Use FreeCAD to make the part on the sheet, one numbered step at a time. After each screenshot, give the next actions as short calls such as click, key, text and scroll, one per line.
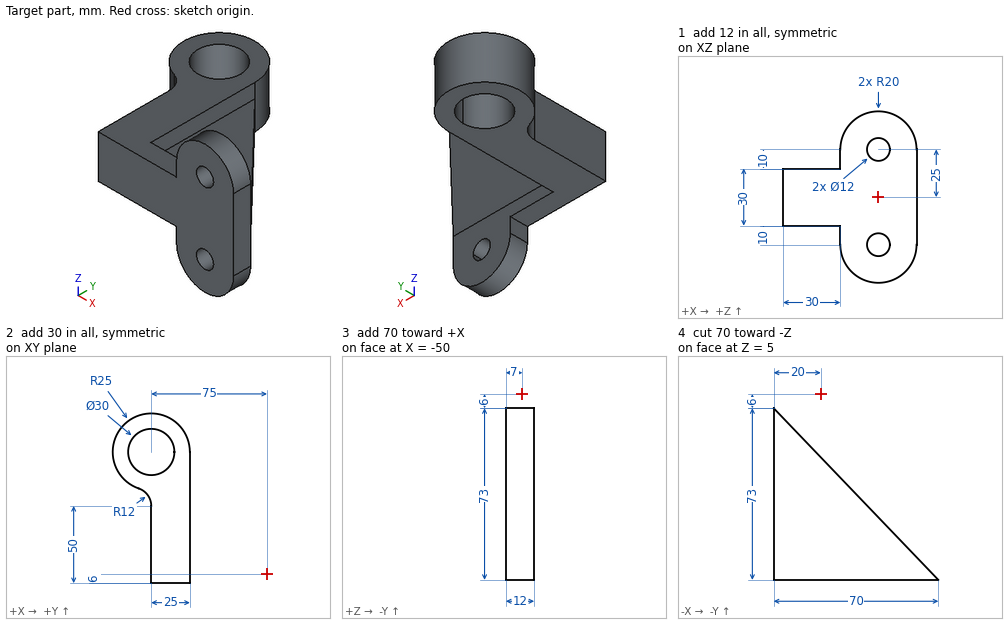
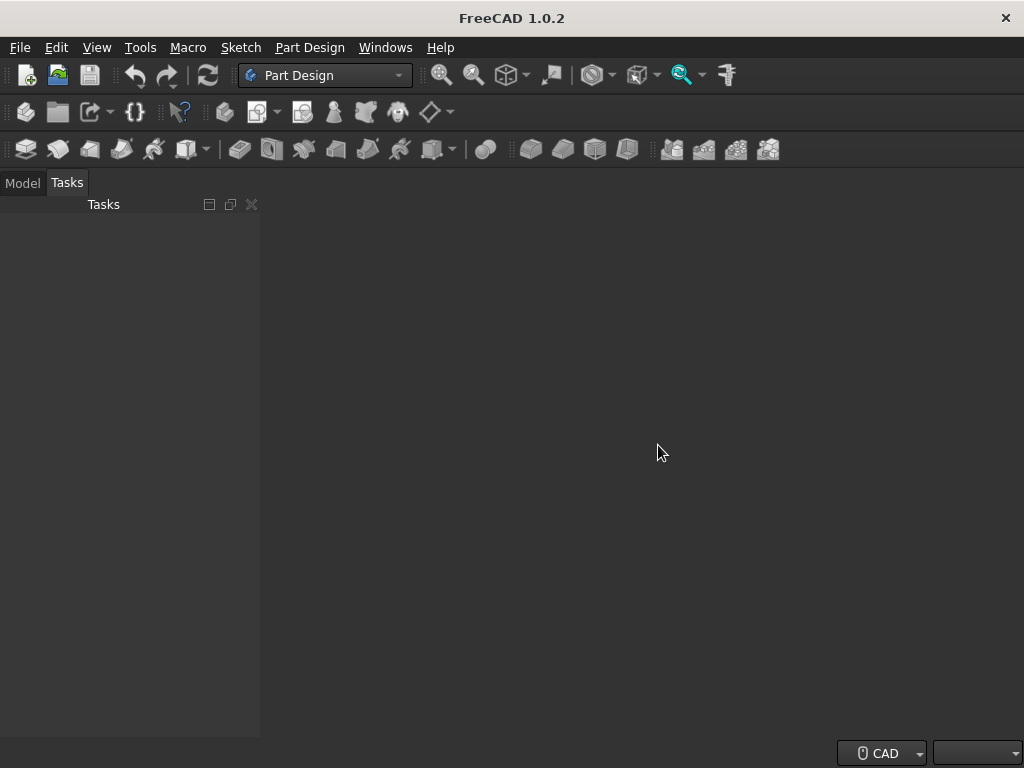
click(26, 76)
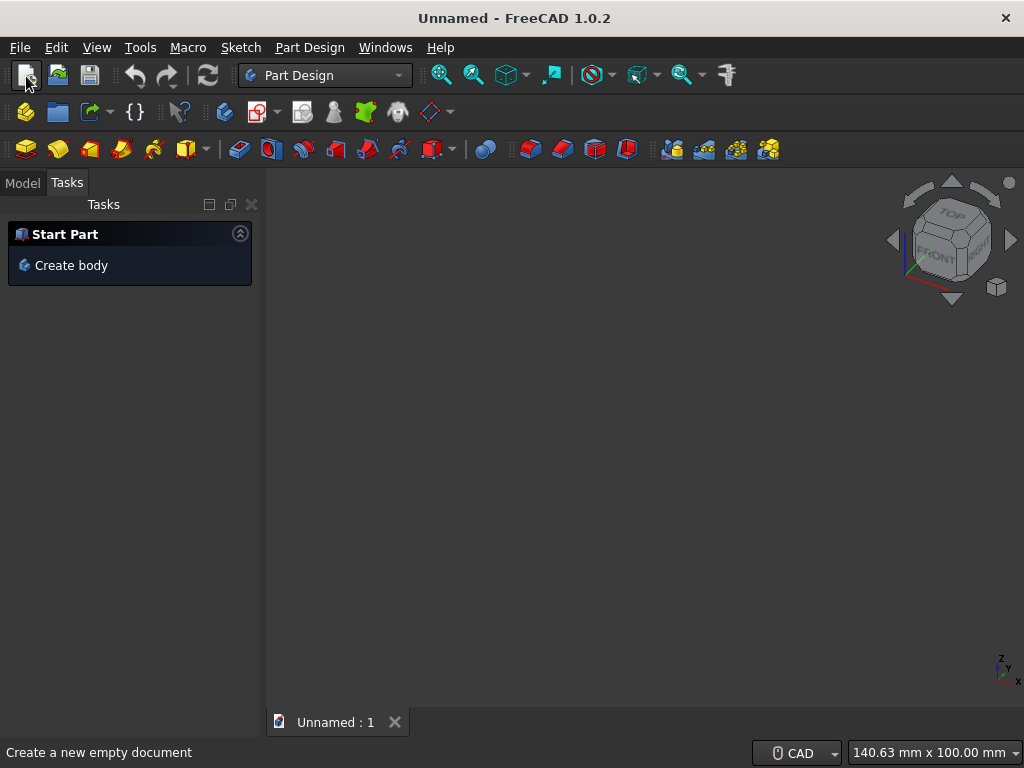
click(258, 112)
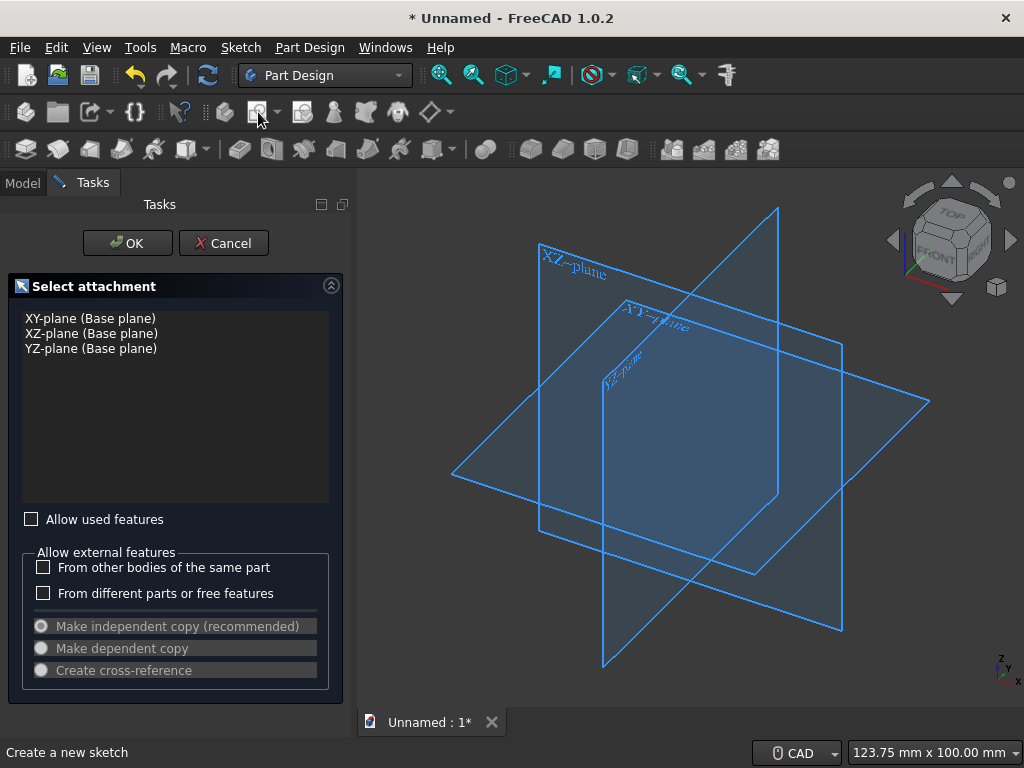
click(82, 334)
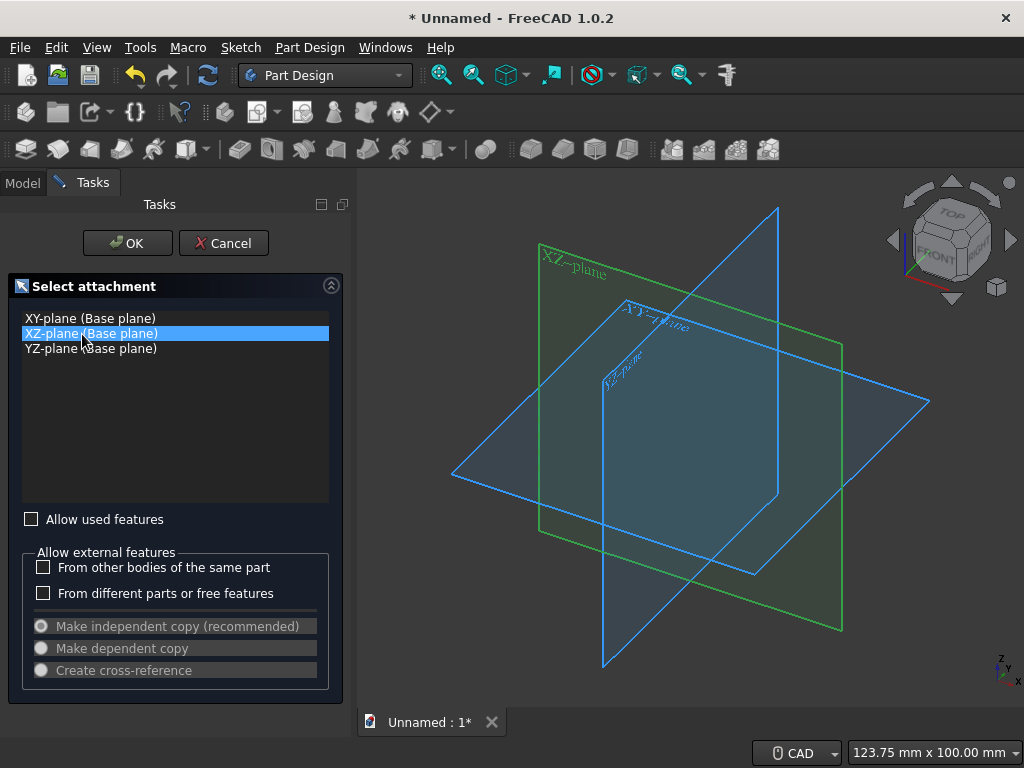
click(128, 243)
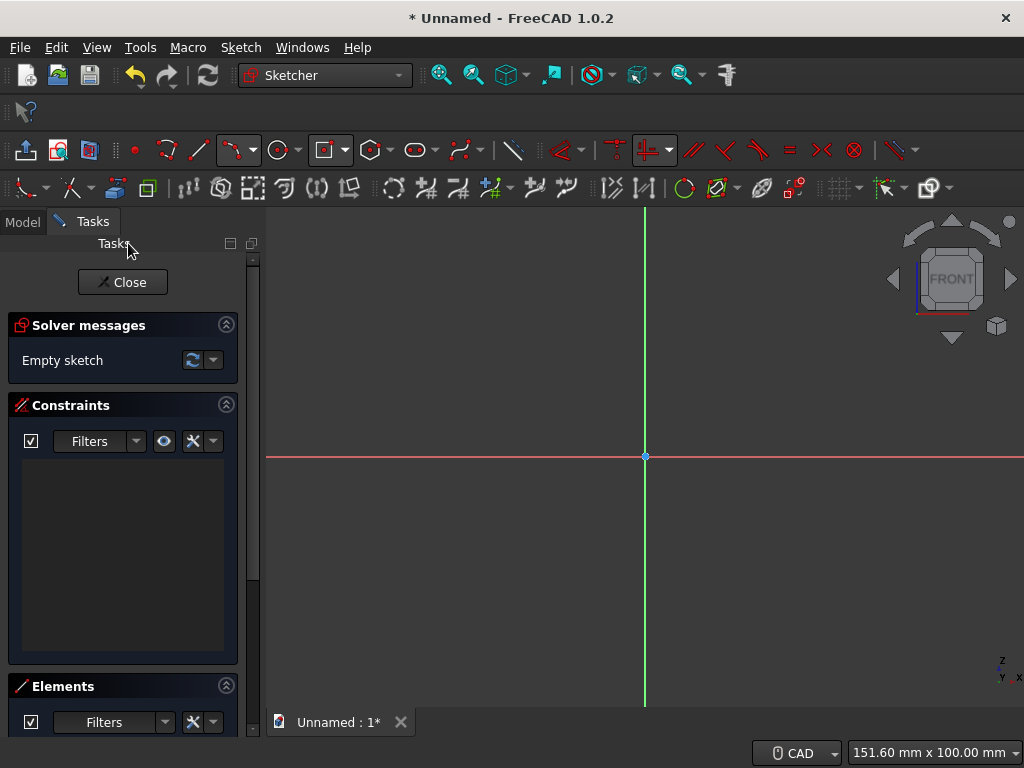
scroll(590, 457, down, 2)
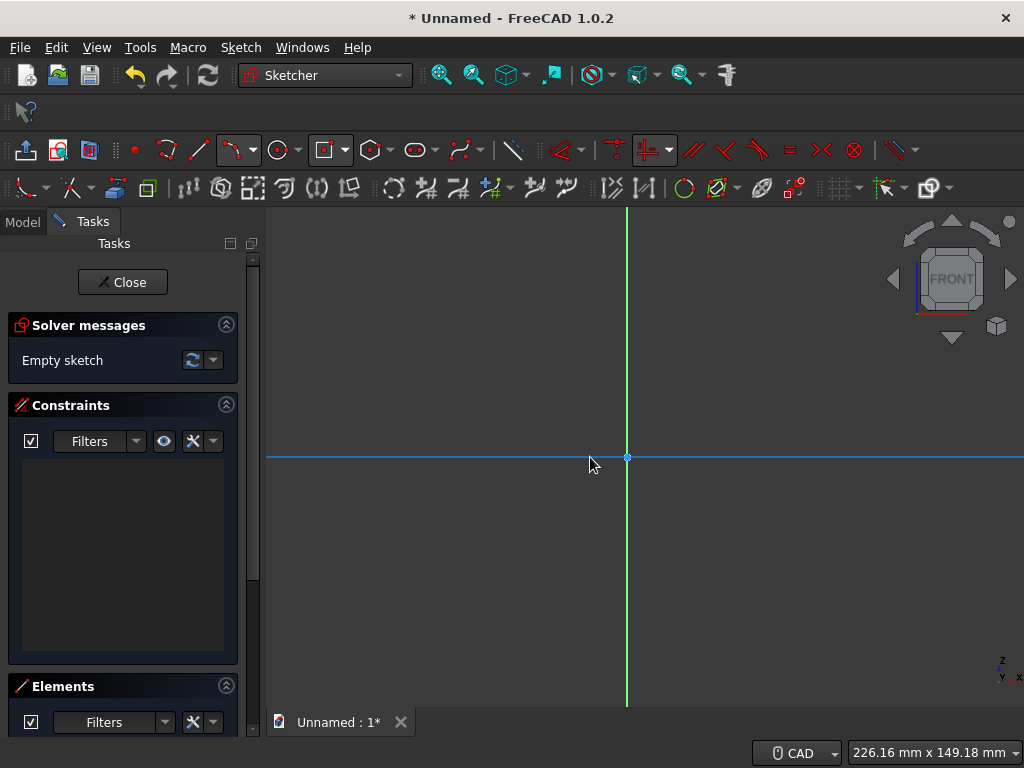
click(168, 150)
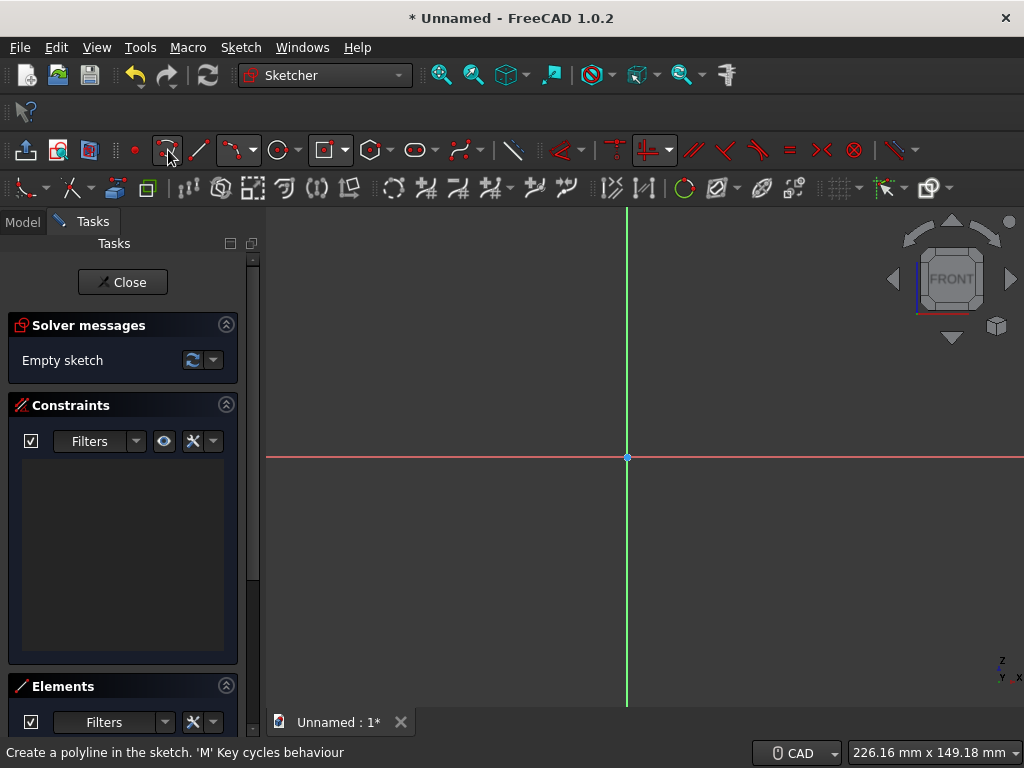
click(560, 541)
click(560, 507)
click(459, 507)
click(459, 407)
click(560, 407)
click(560, 373)
right_click(560, 373)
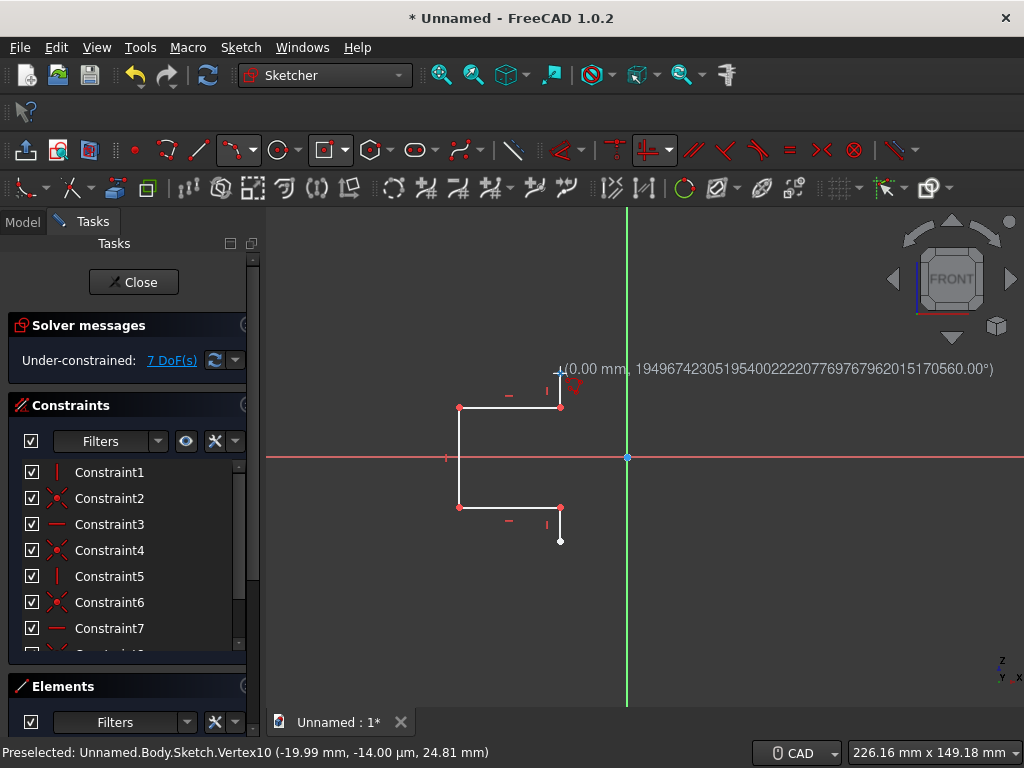
click(200, 150)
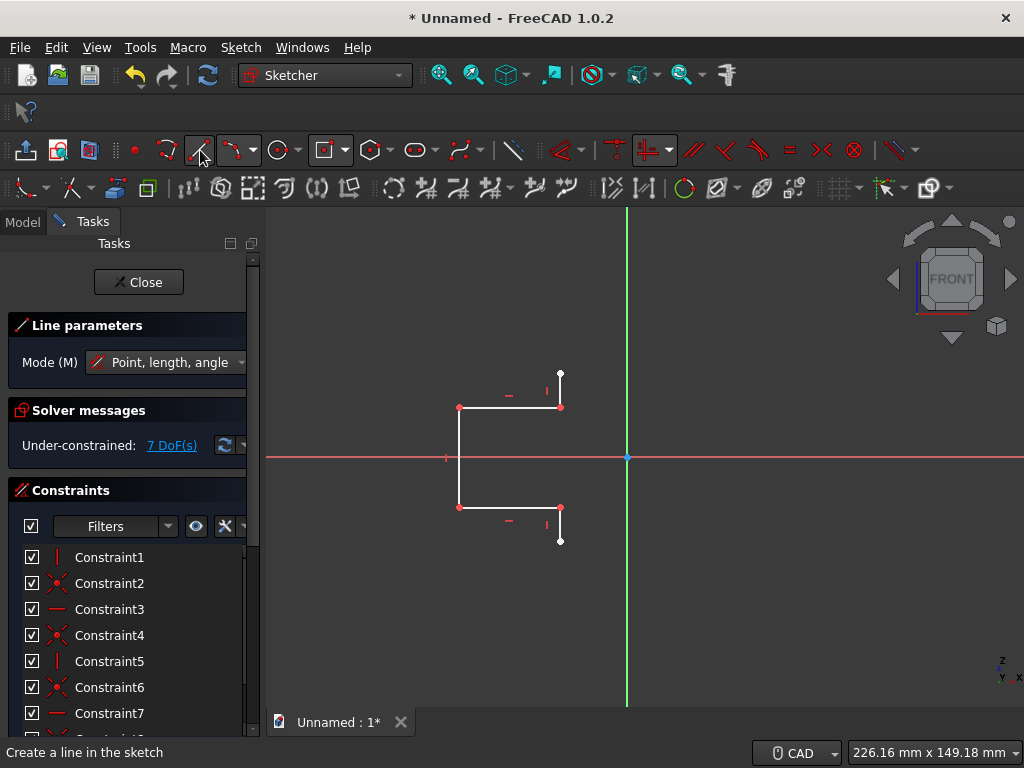
click(694, 373)
click(694, 541)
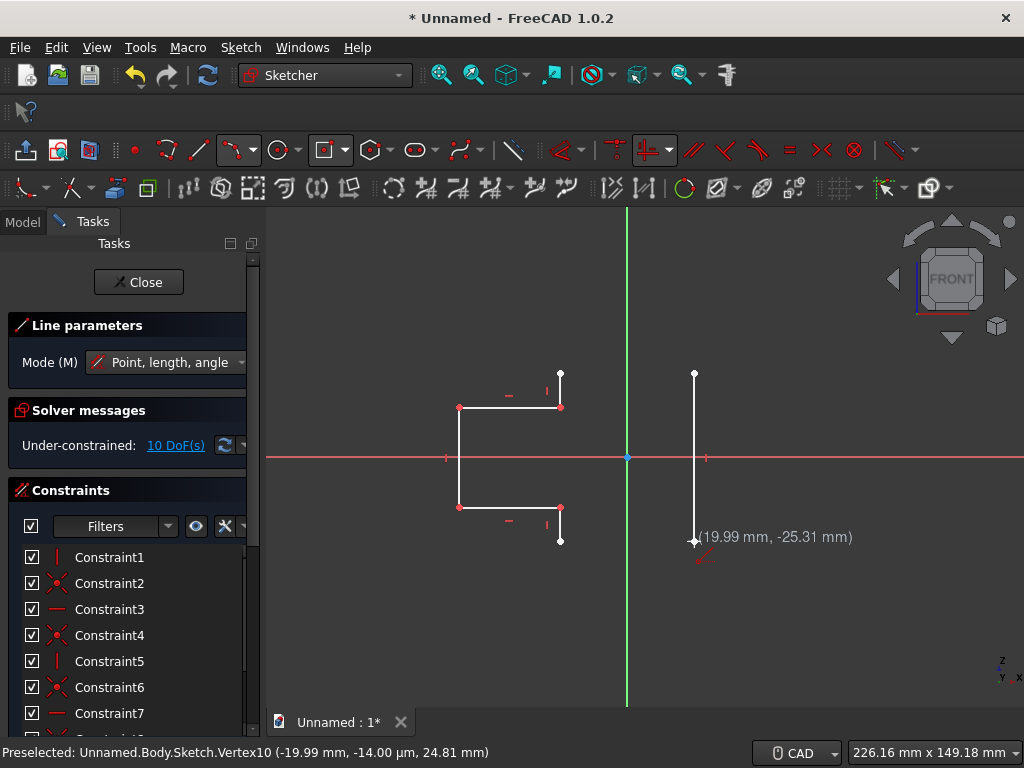
click(232, 150)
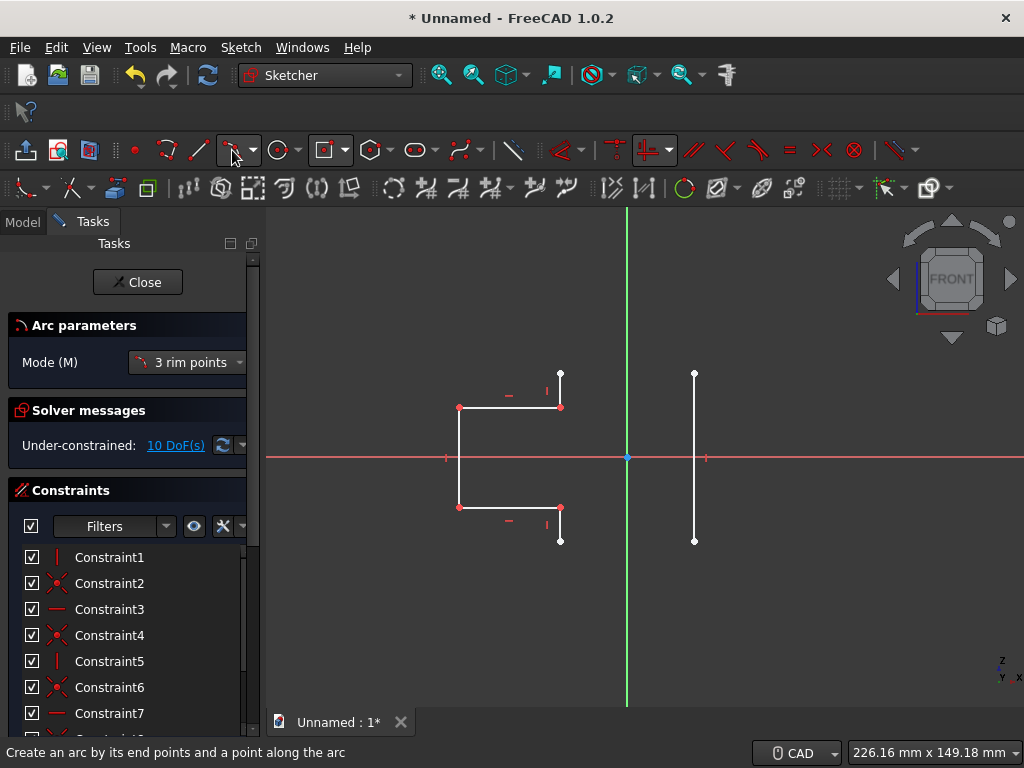
click(560, 374)
click(694, 374)
click(648, 310)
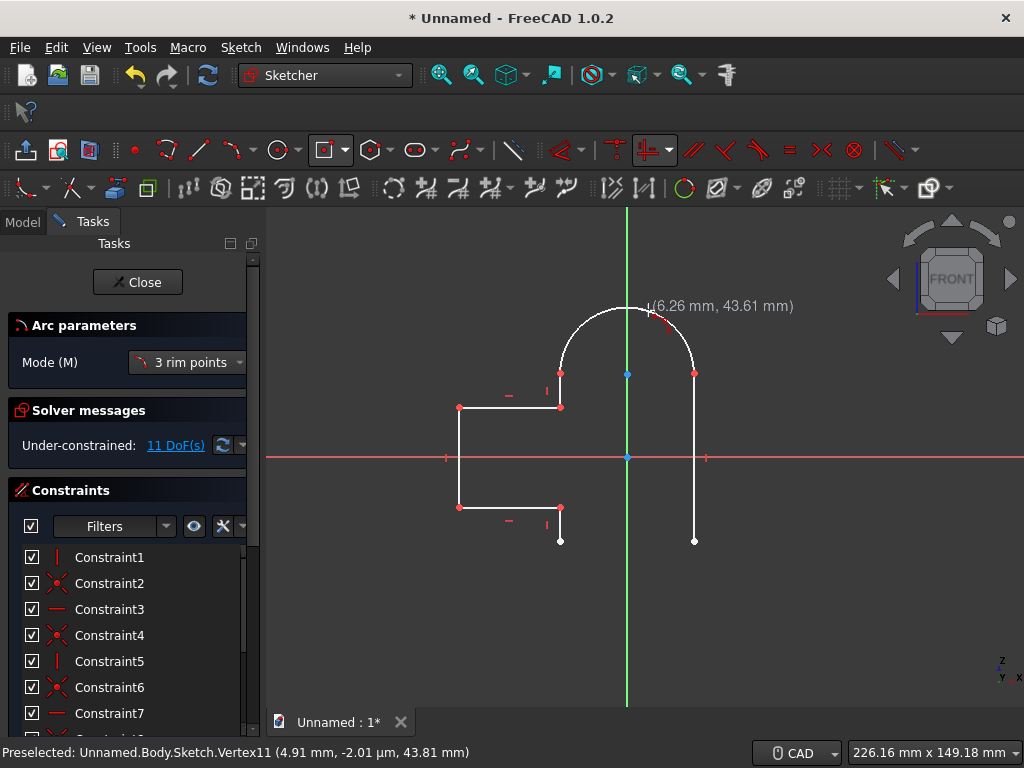
click(694, 542)
click(560, 542)
click(606, 605)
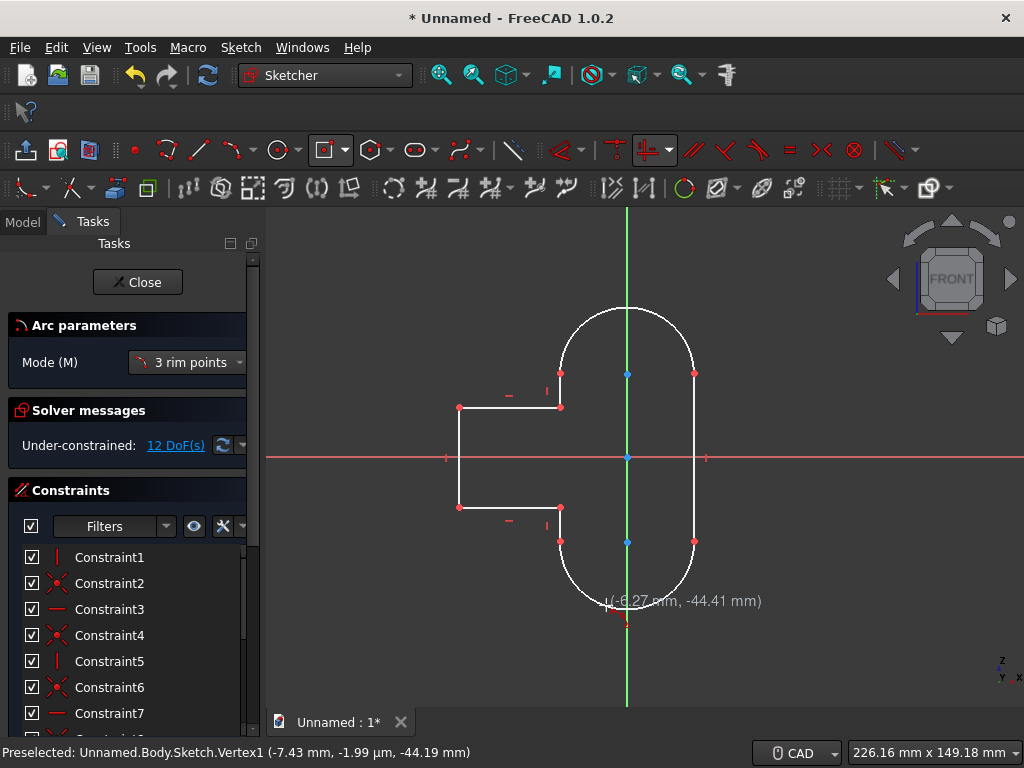
click(278, 150)